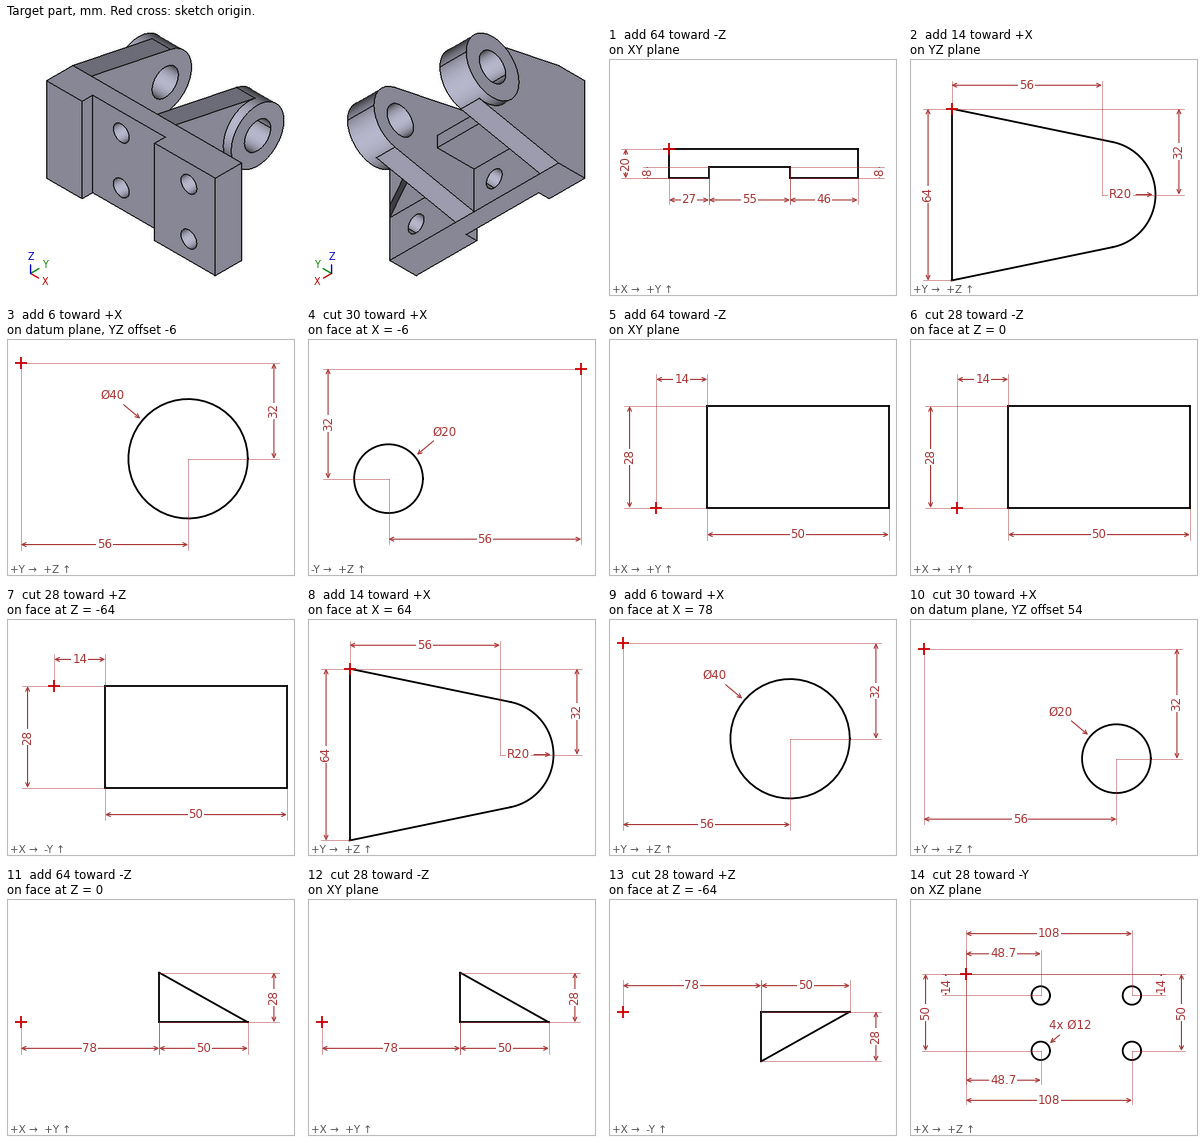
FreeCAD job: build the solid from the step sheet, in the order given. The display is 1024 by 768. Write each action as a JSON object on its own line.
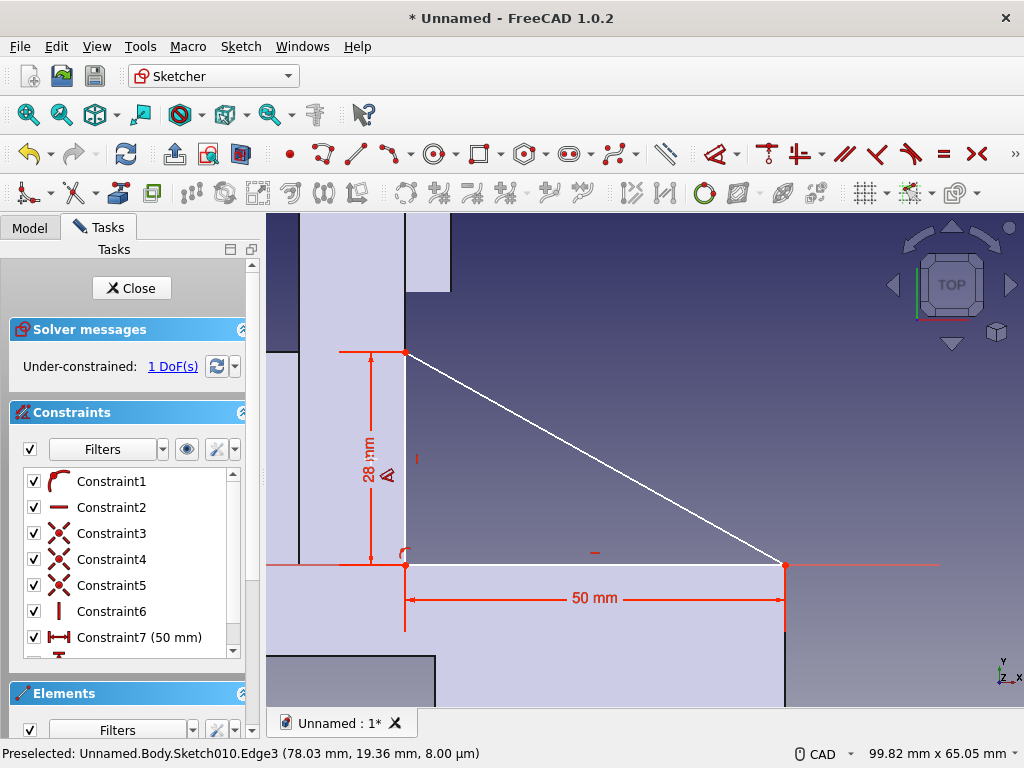
{"action": "left_click", "coordinate": [405, 565]}
{"action": "left_click", "coordinate": [350, 599]}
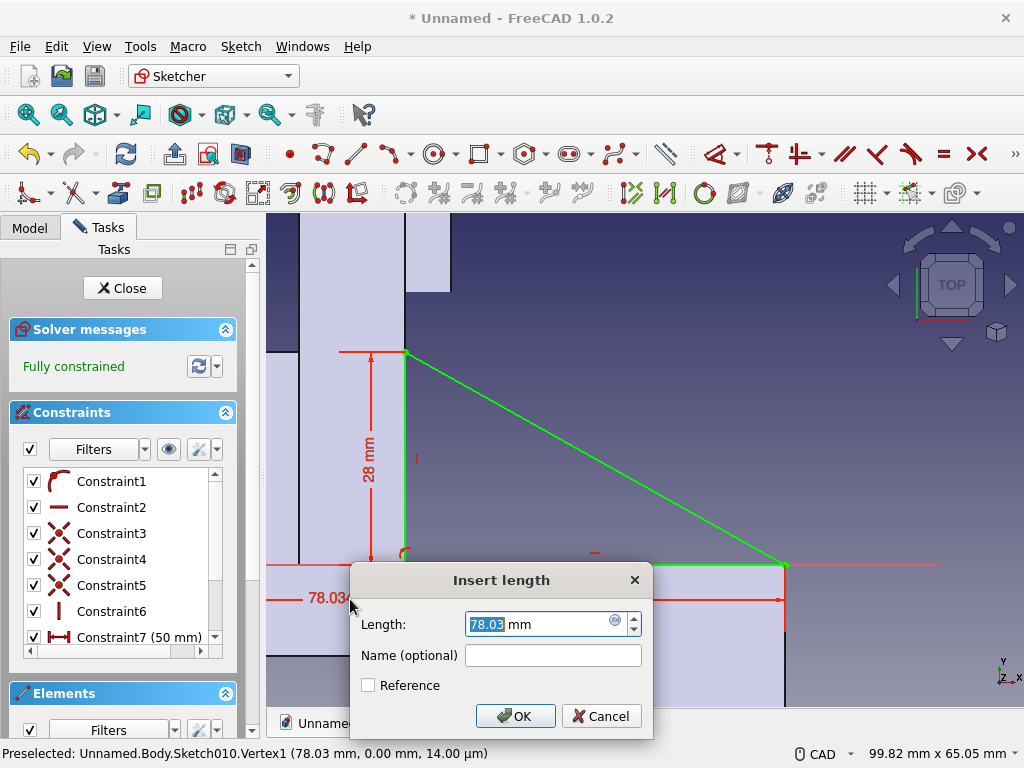
{"action": "type", "text": "78"}
{"action": "key", "text": "Return"}
{"action": "key", "text": "Escape"}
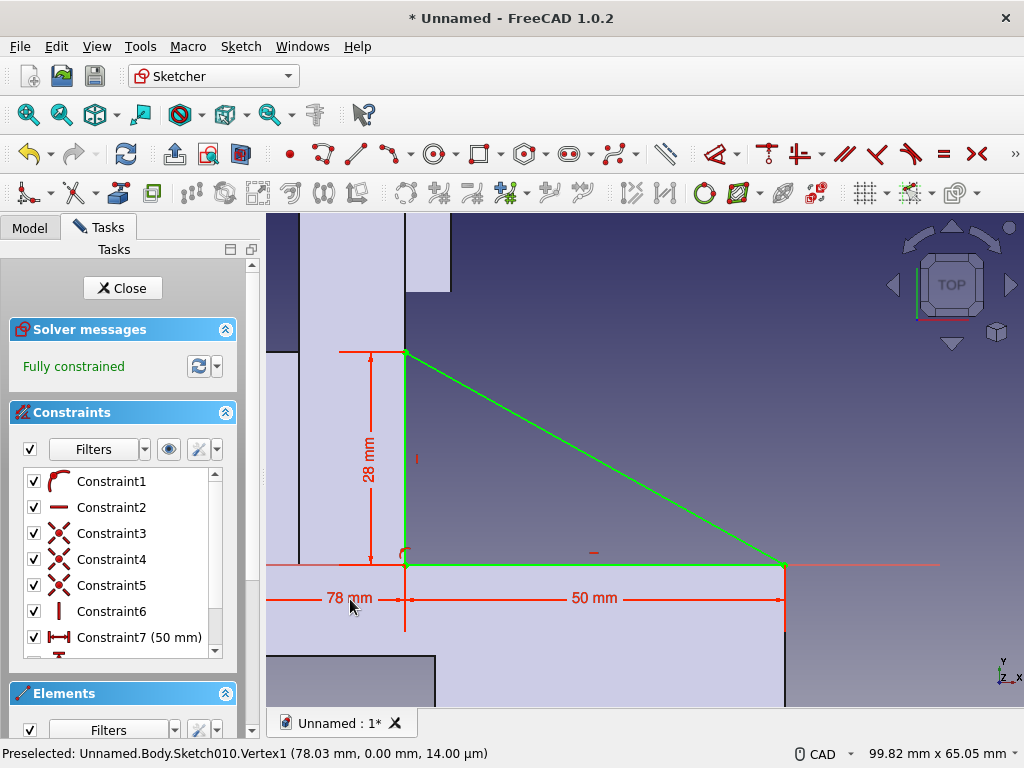
{"action": "left_click", "coordinate": [123, 288]}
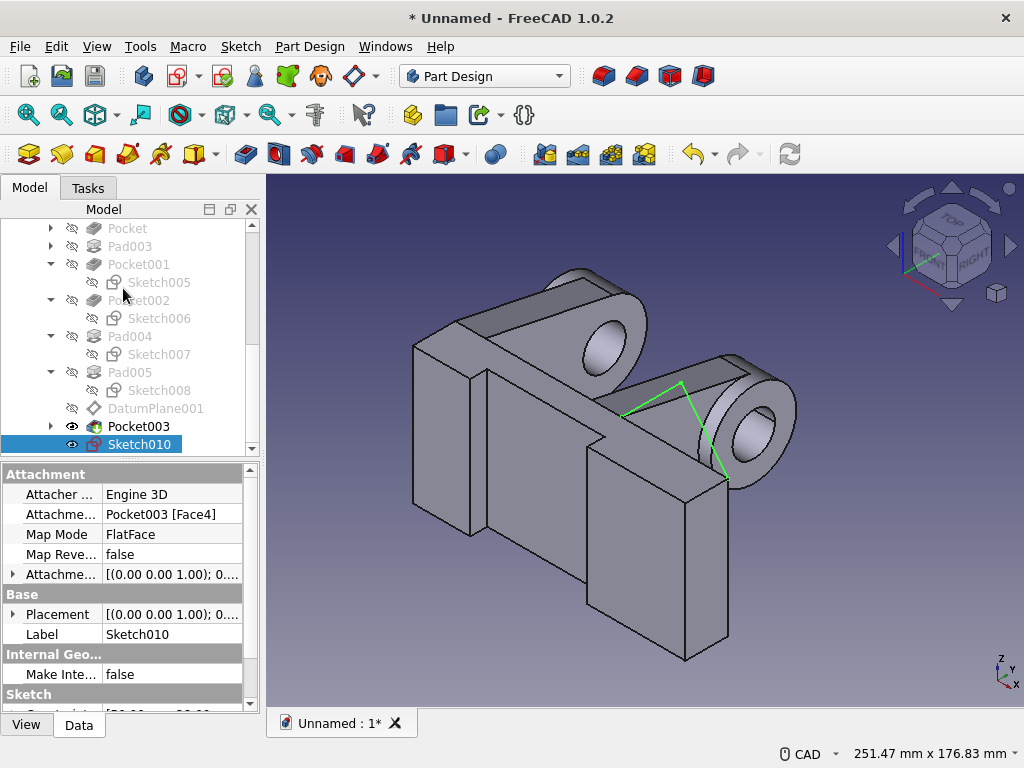
{"action": "left_click", "coordinate": [29, 154]}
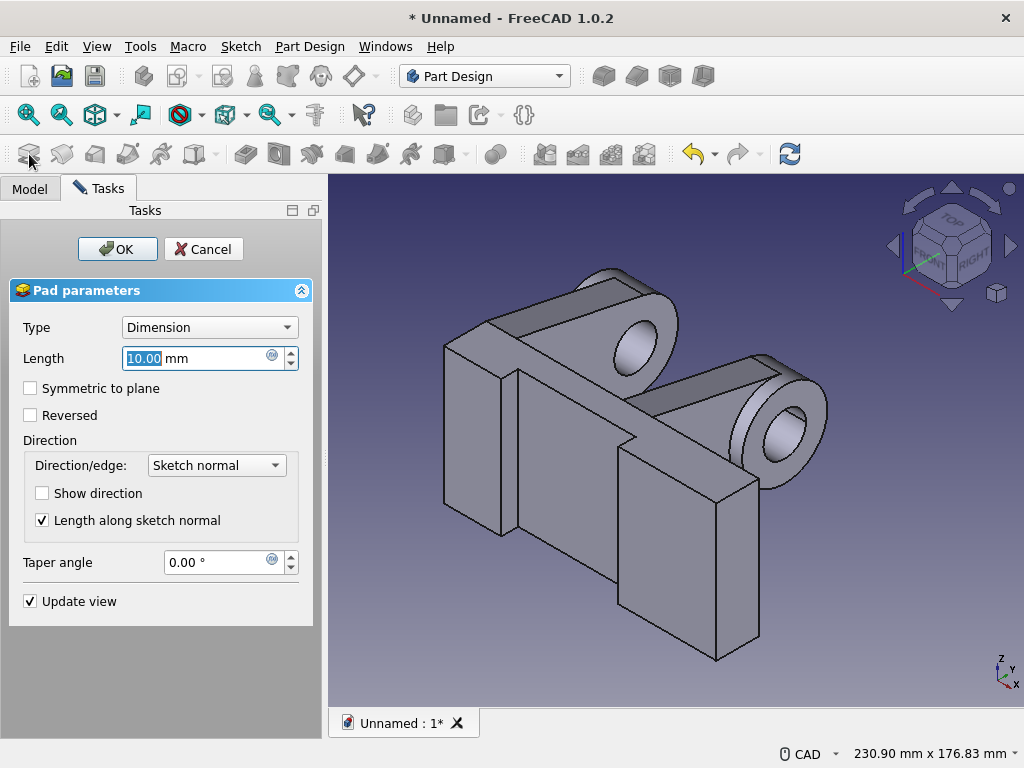
{"action": "type", "text": "64"}
{"action": "key", "text": "Tab"}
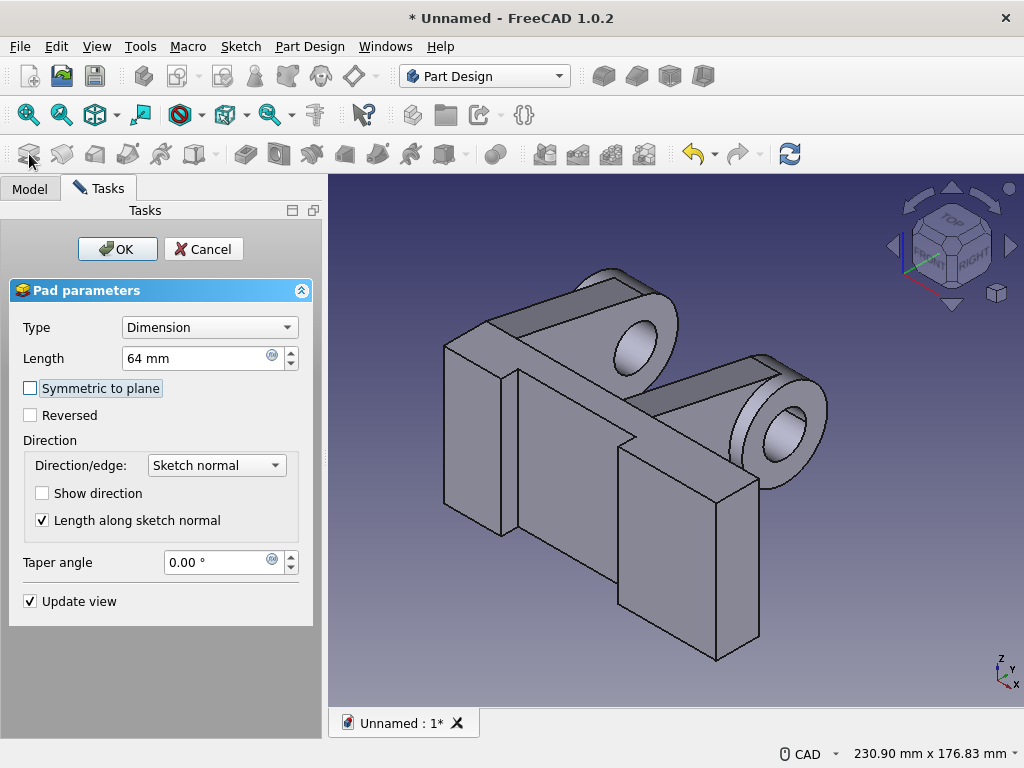
{"action": "left_click", "coordinate": [31, 415]}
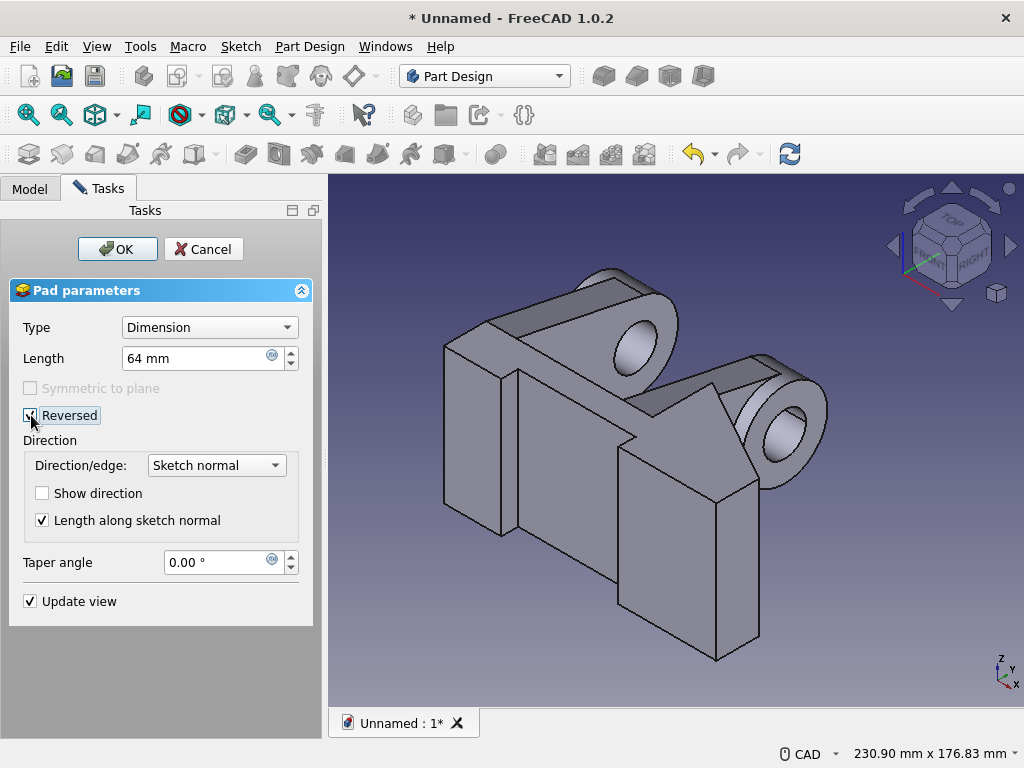
{"action": "left_click", "coordinate": [118, 249]}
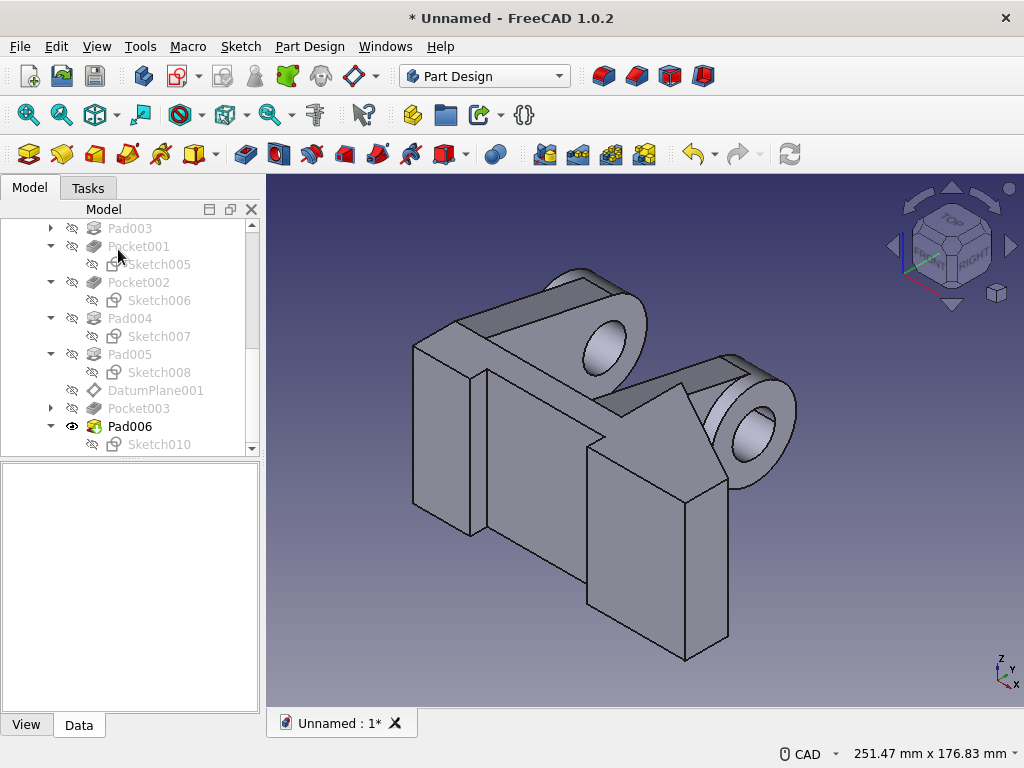
{"action": "left_click", "coordinate": [176, 76]}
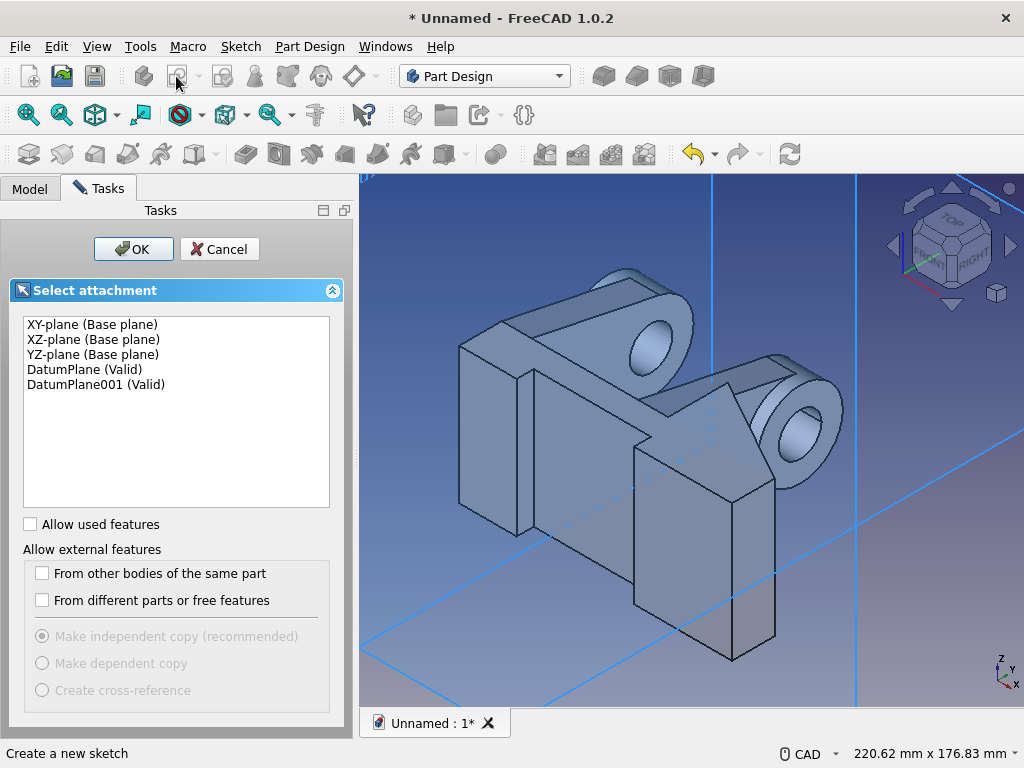
{"action": "left_click", "coordinate": [84, 324]}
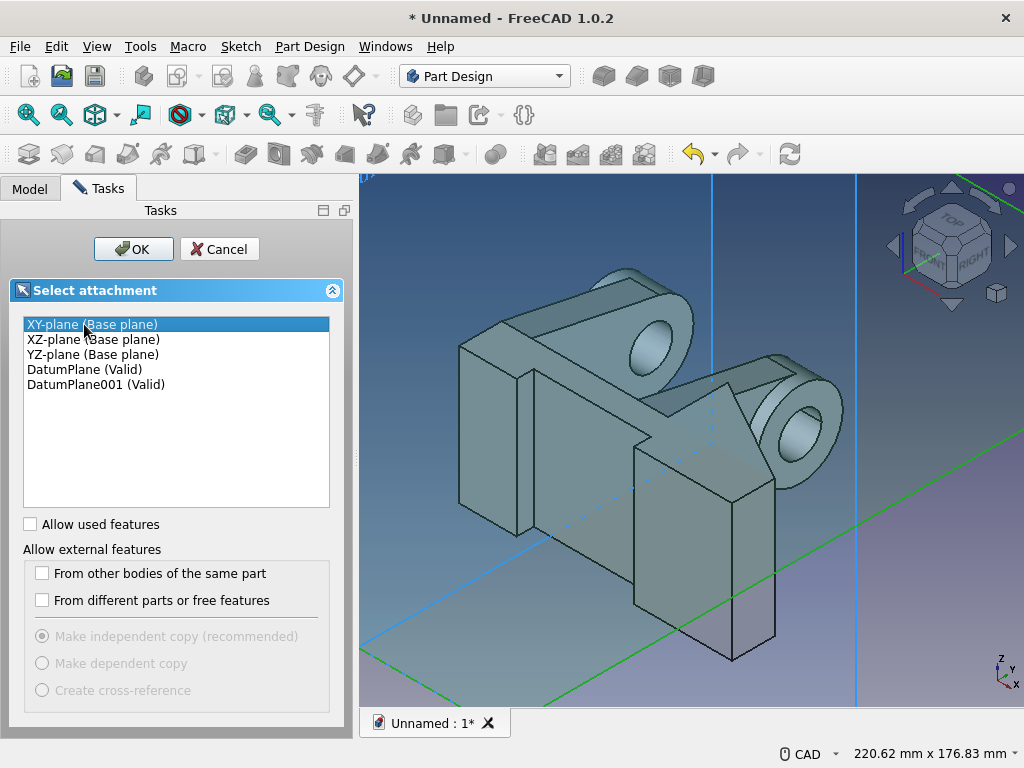
{"action": "left_click", "coordinate": [134, 249]}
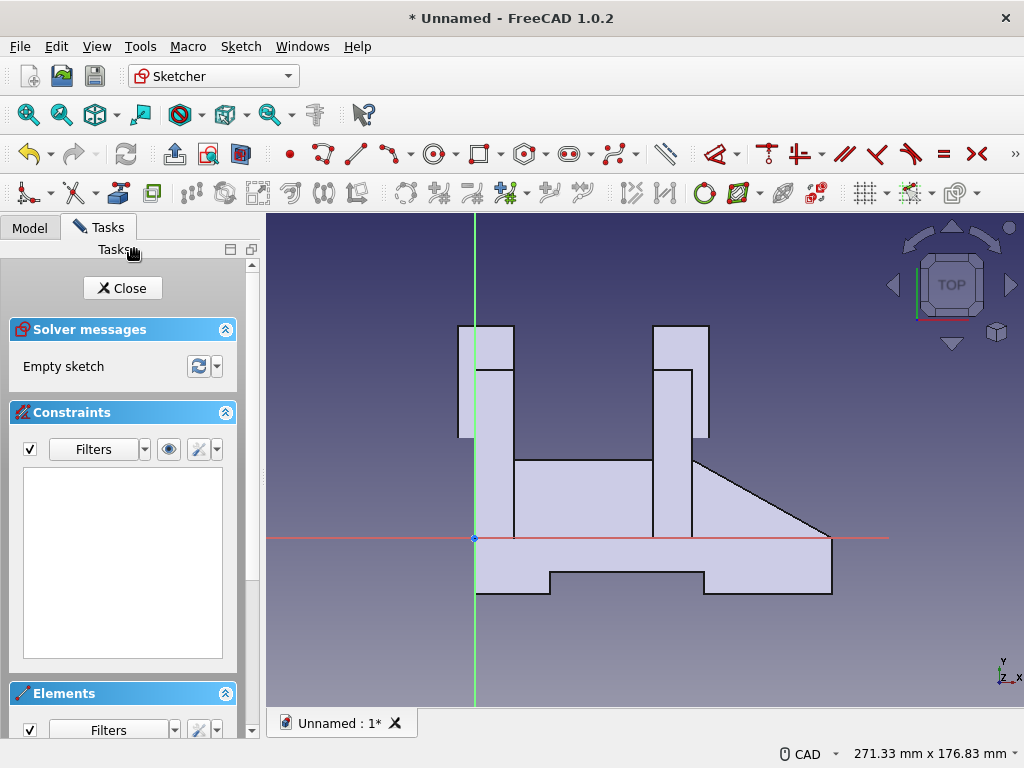
{"action": "scroll", "coordinate": [859, 522], "scroll_direction": "up", "scroll_amount": 5}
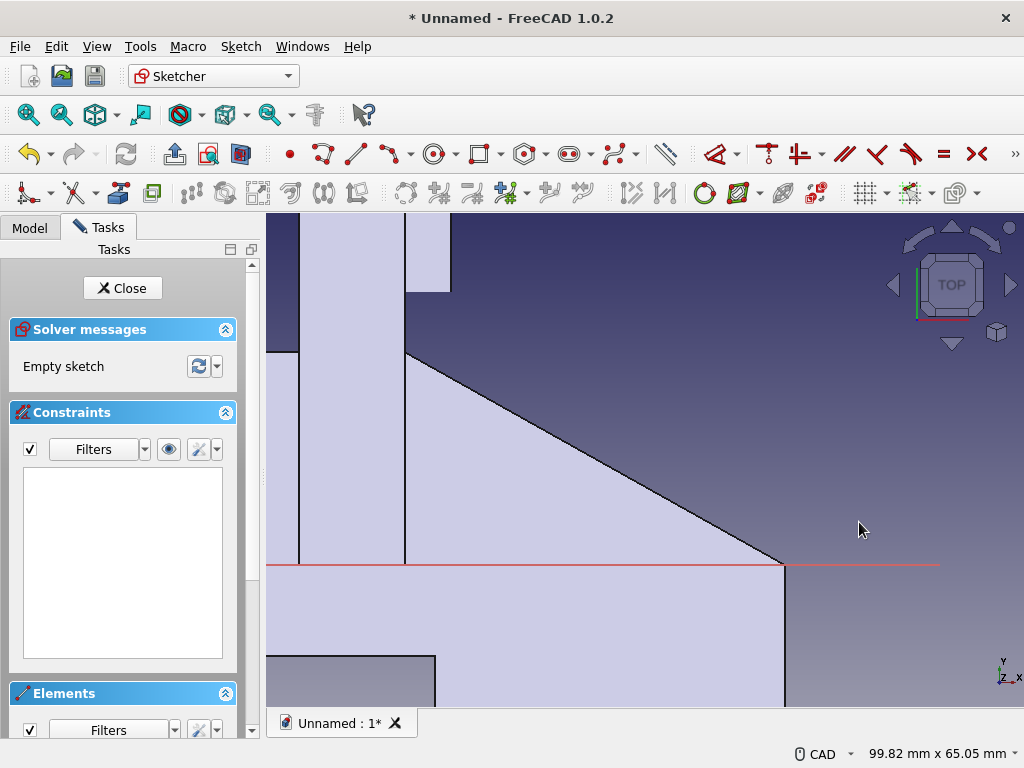
{"action": "left_click", "coordinate": [323, 154]}